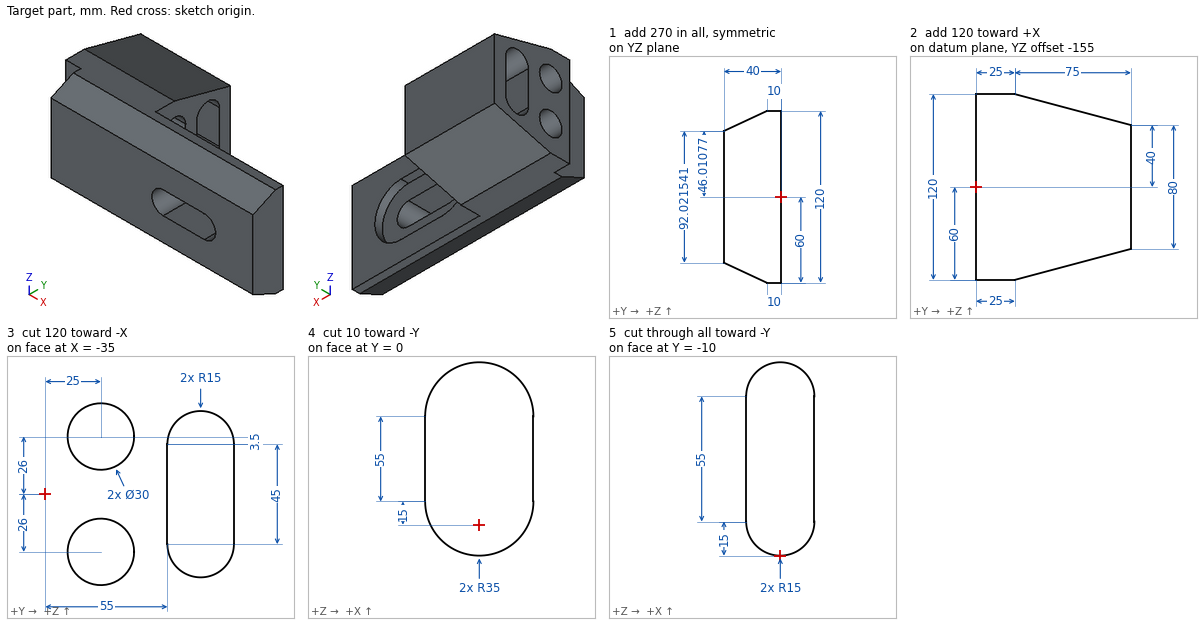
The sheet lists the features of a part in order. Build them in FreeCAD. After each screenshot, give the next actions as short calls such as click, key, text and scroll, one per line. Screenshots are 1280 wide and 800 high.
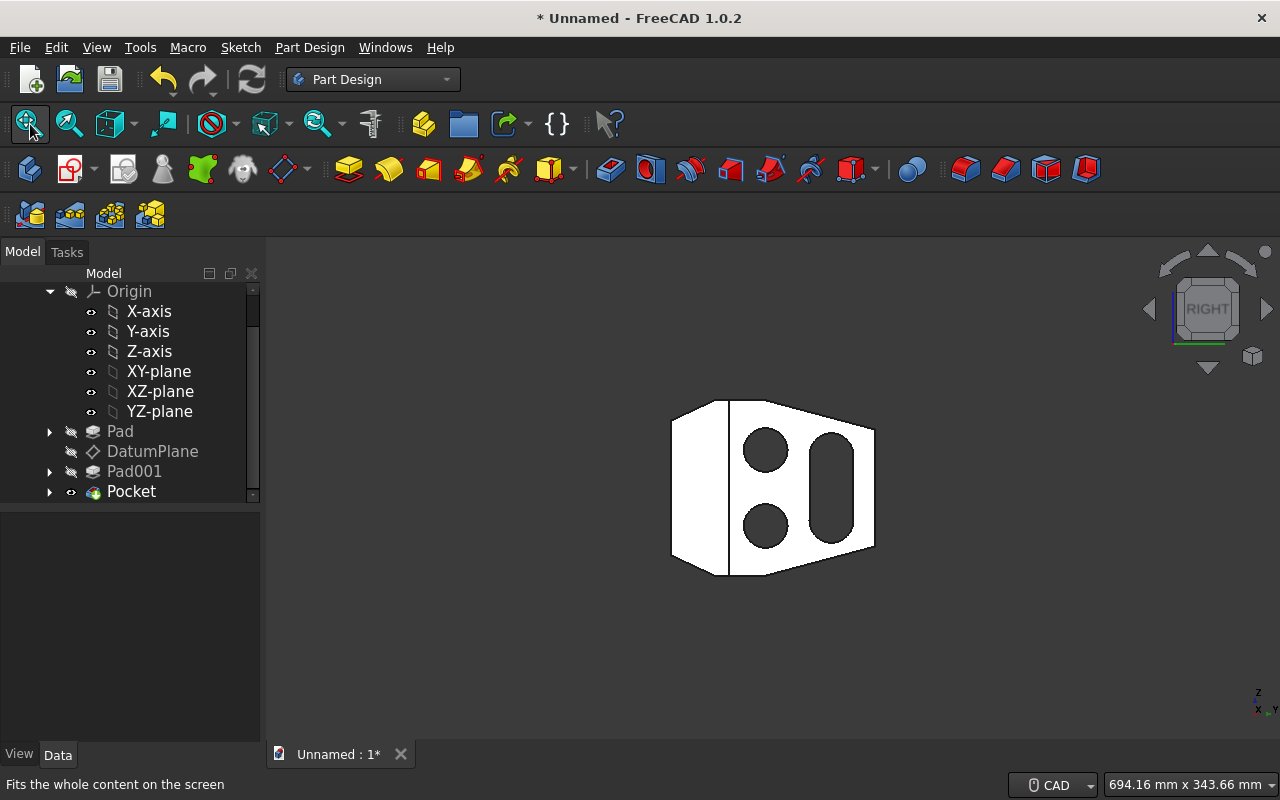
key(4)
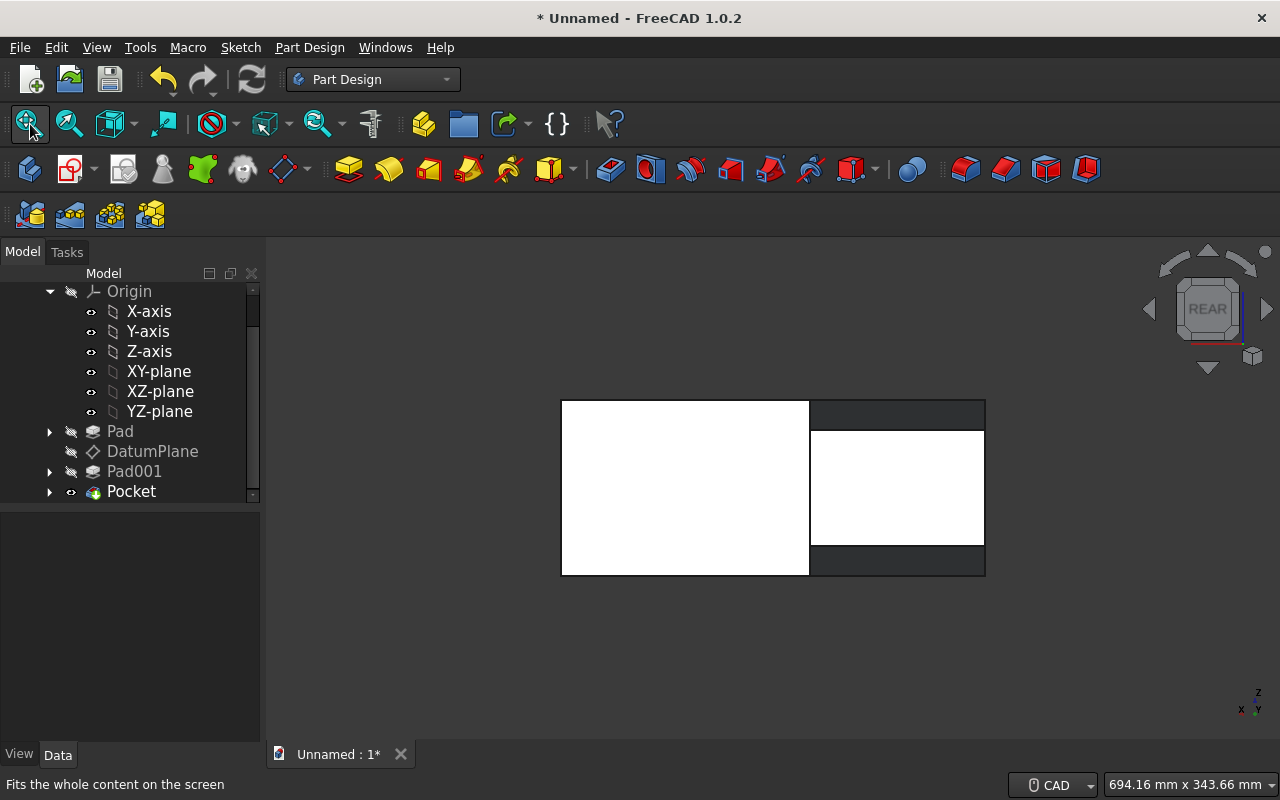
click(30, 124)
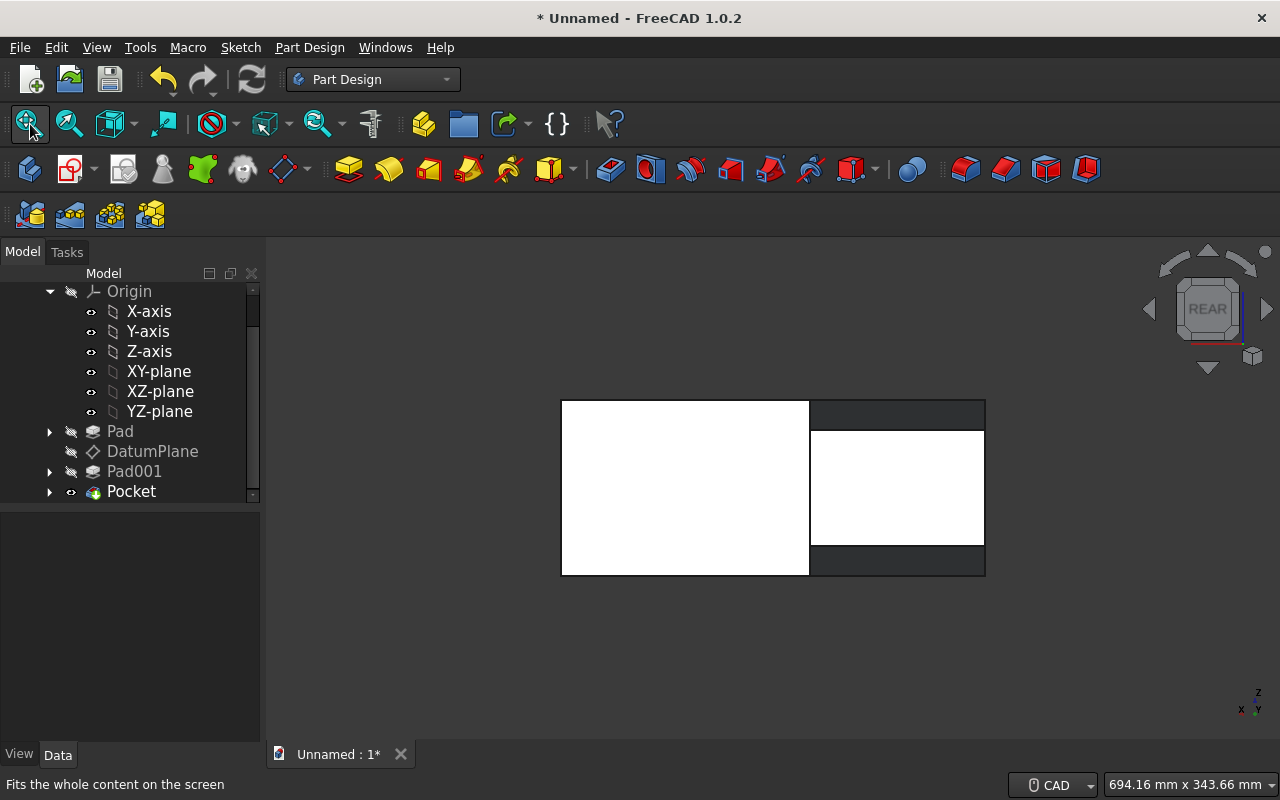
click(685, 487)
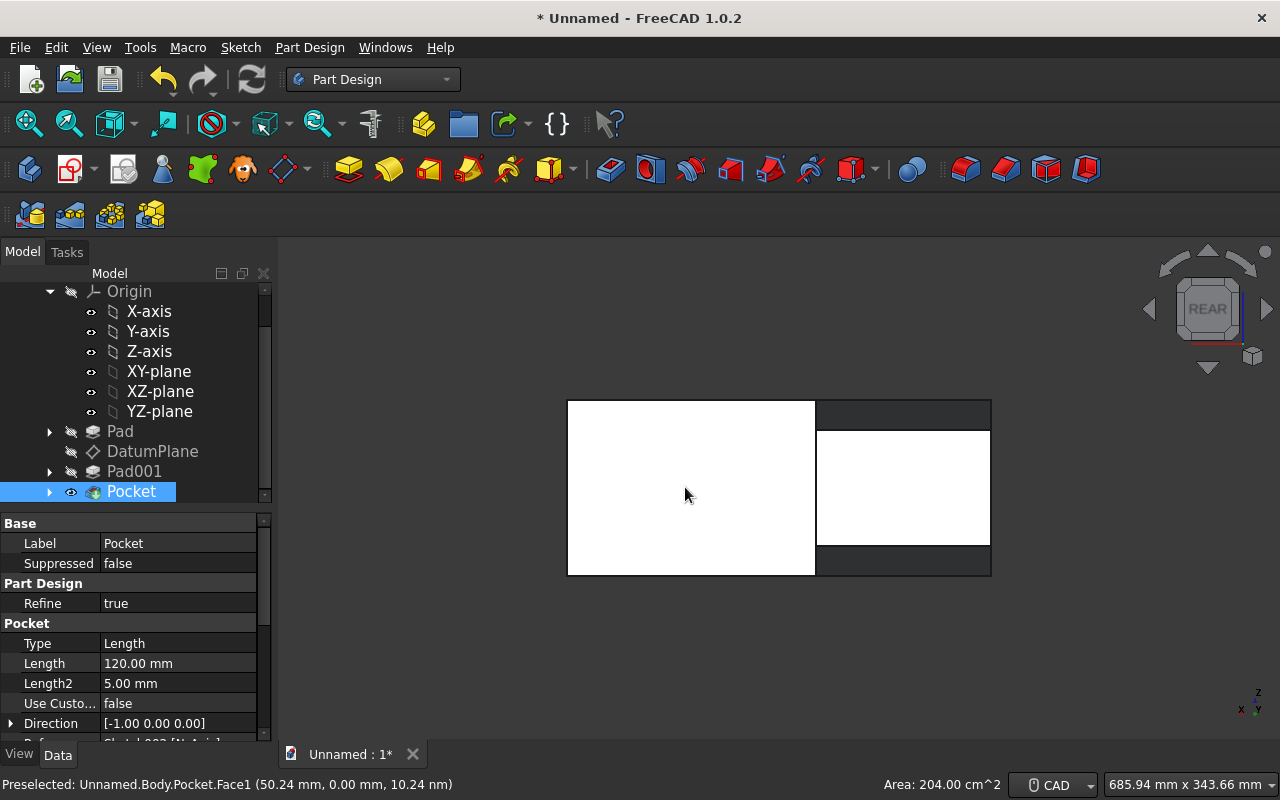
click(70, 170)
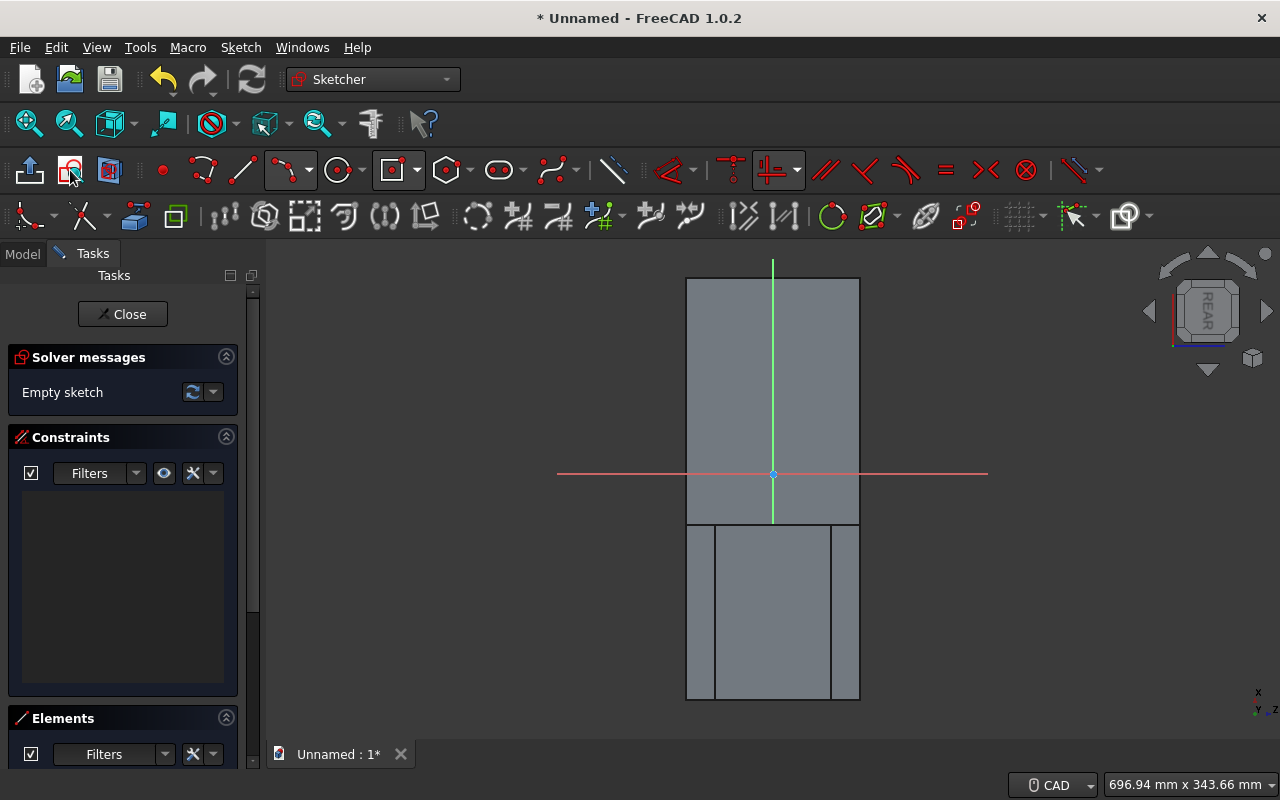
click(110, 170)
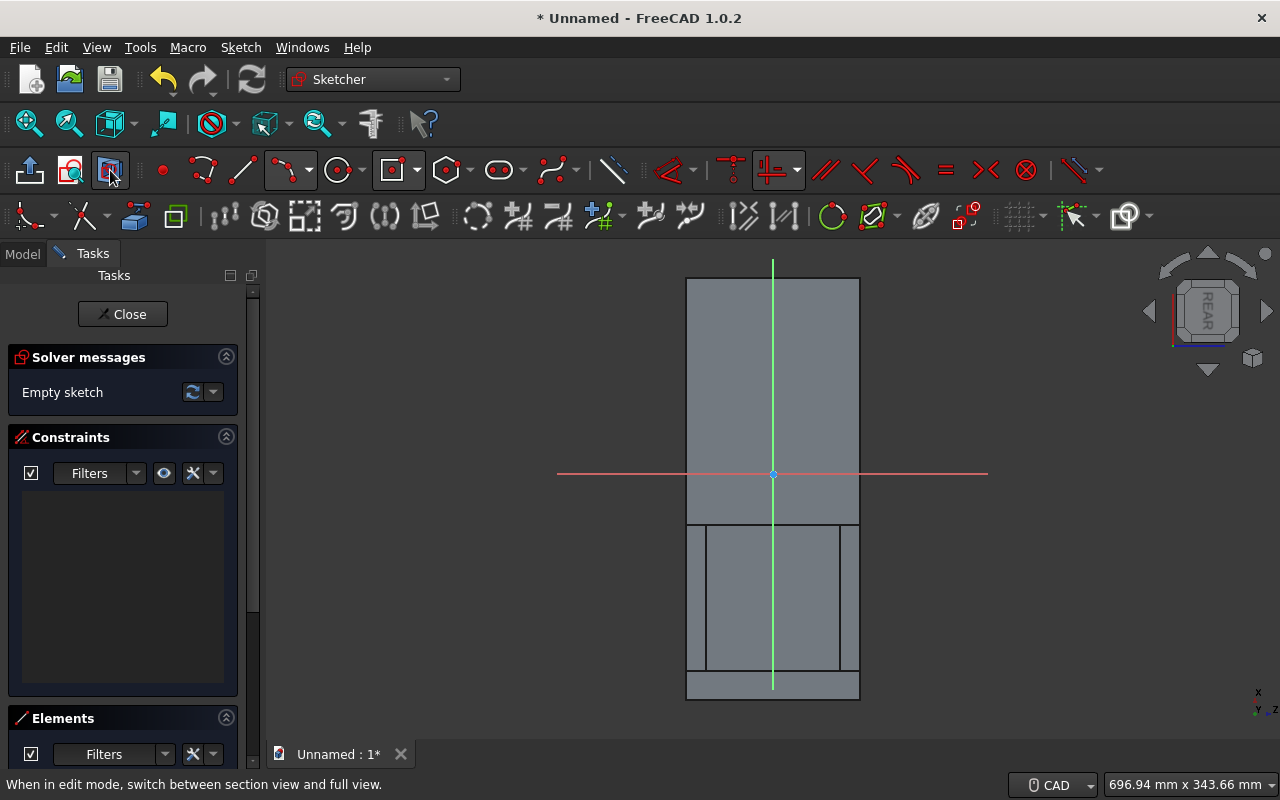
scroll(856, 320, up, 3)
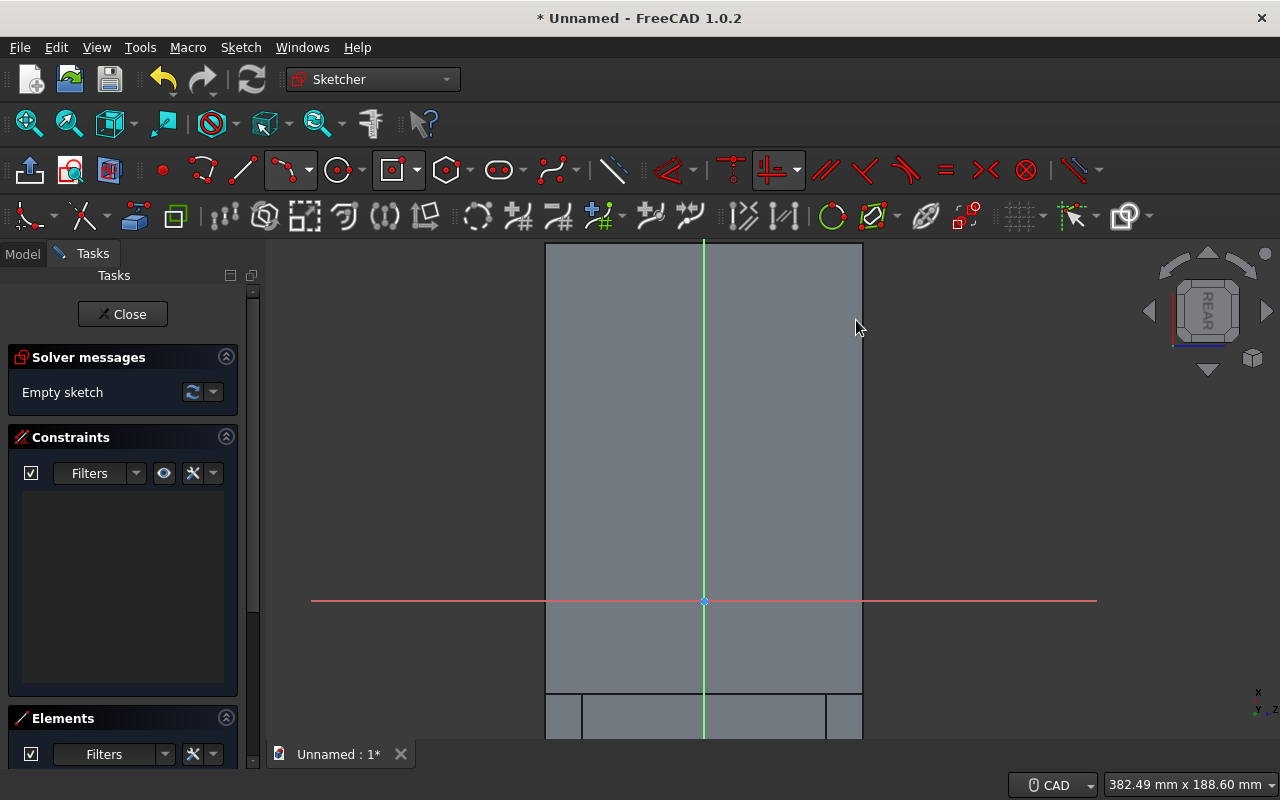
click(500, 170)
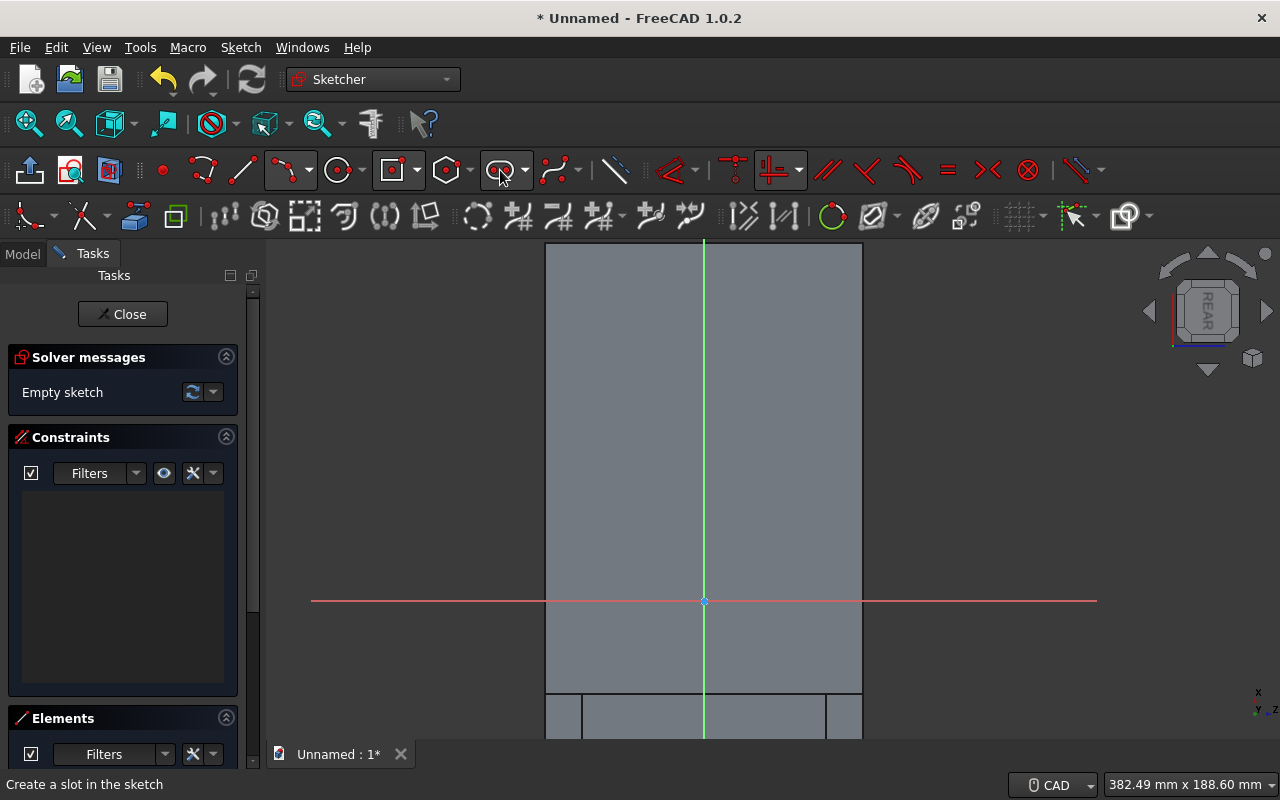
click(704, 562)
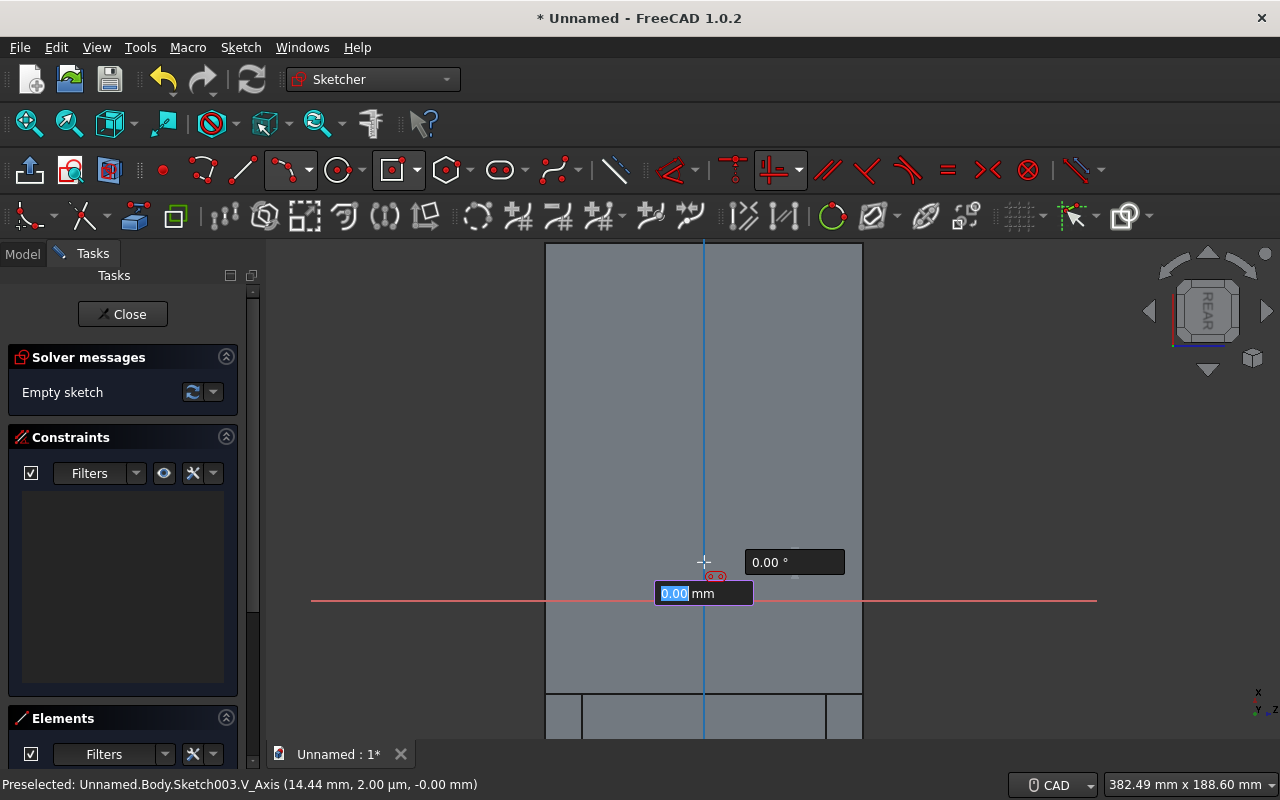
click(713, 416)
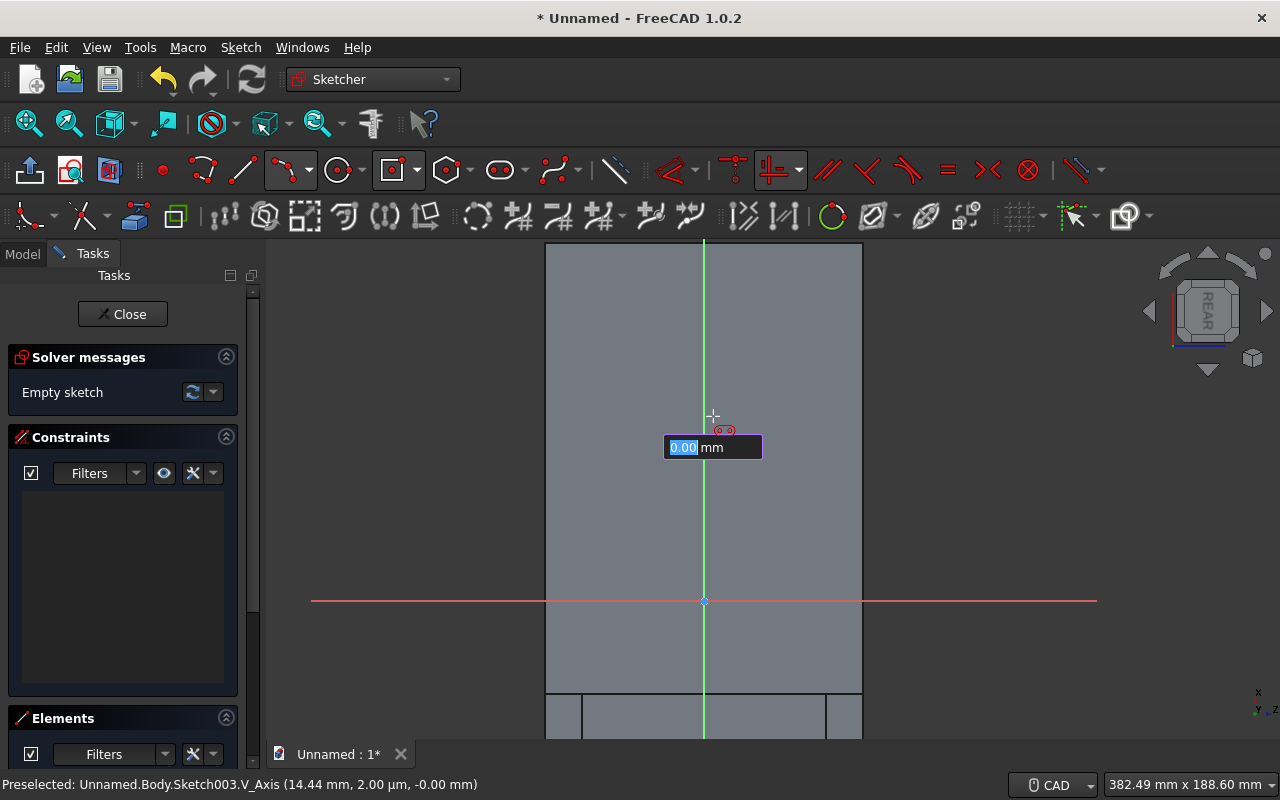
click(611, 489)
key(Escape)